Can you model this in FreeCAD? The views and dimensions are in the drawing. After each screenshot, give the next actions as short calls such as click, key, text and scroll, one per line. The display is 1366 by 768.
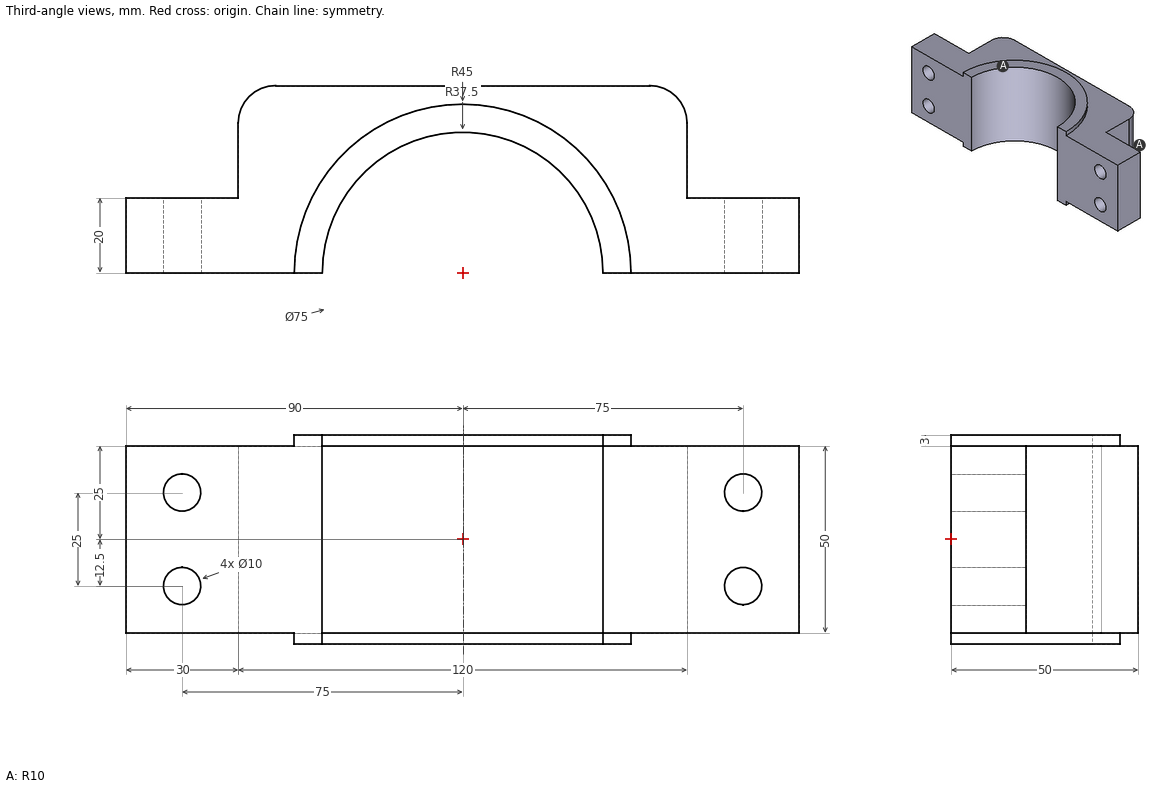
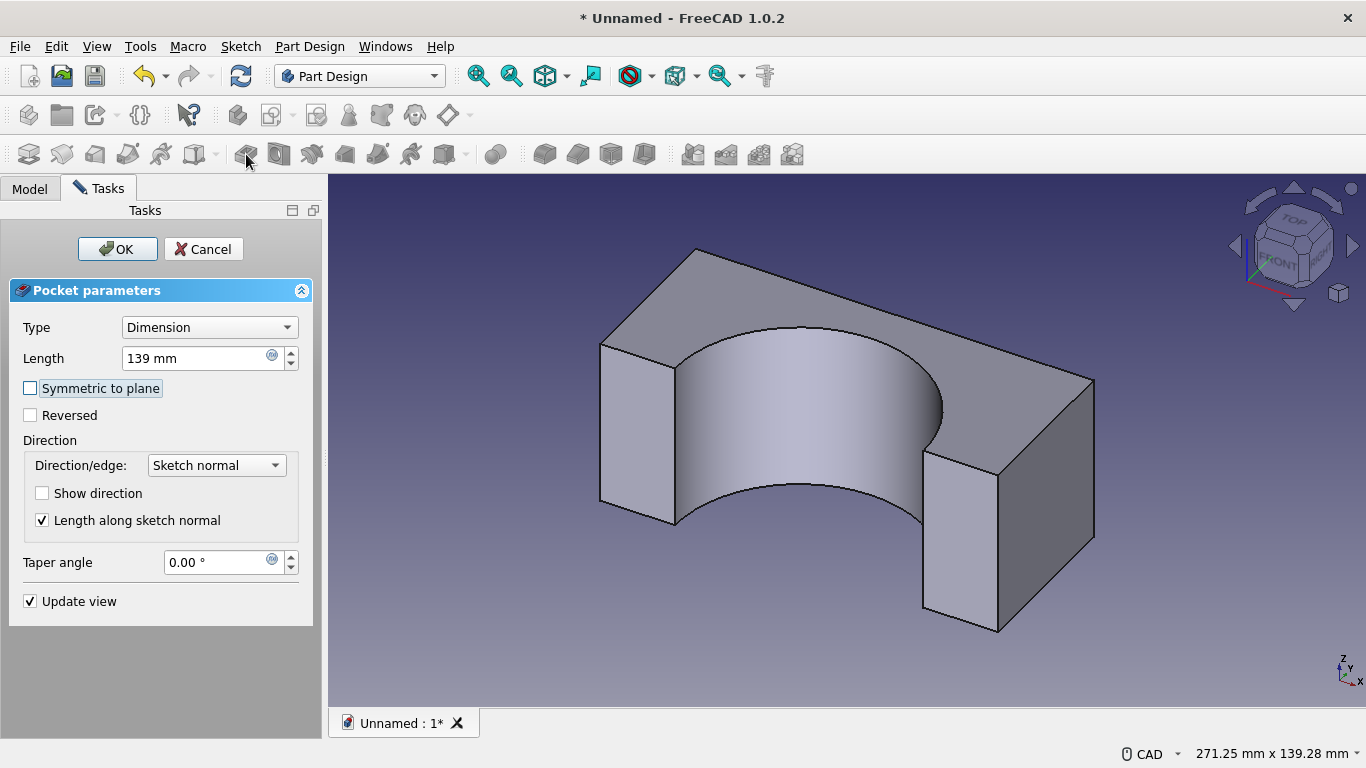
click(118, 249)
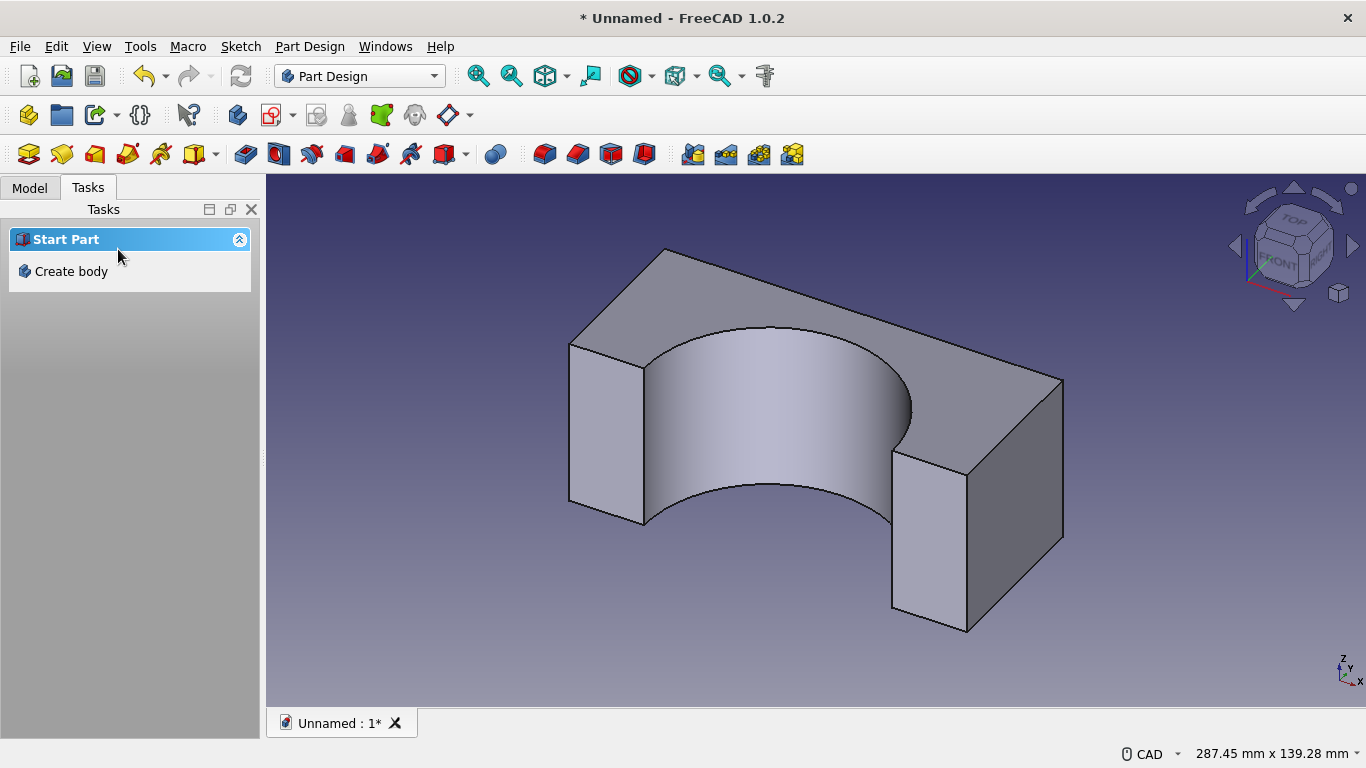
key(0)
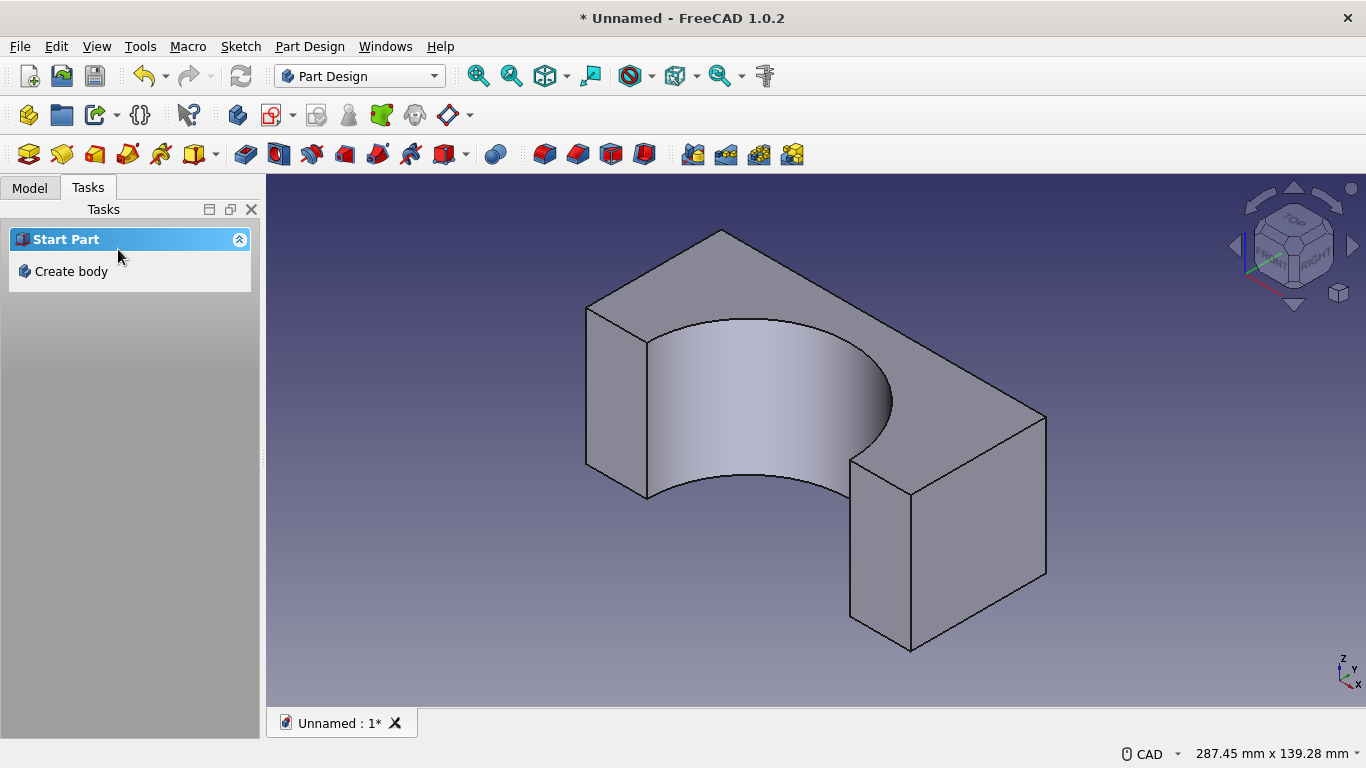
key(2)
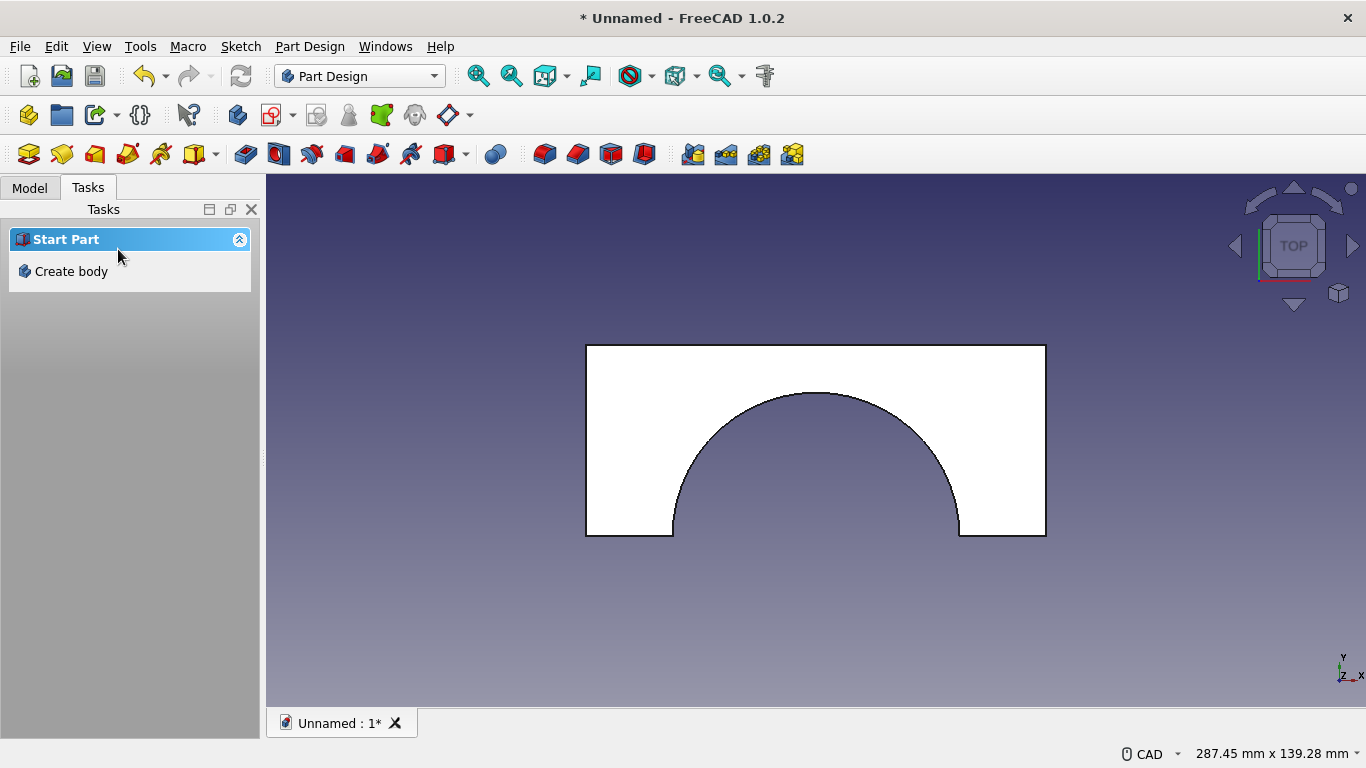
key(v)
key(f)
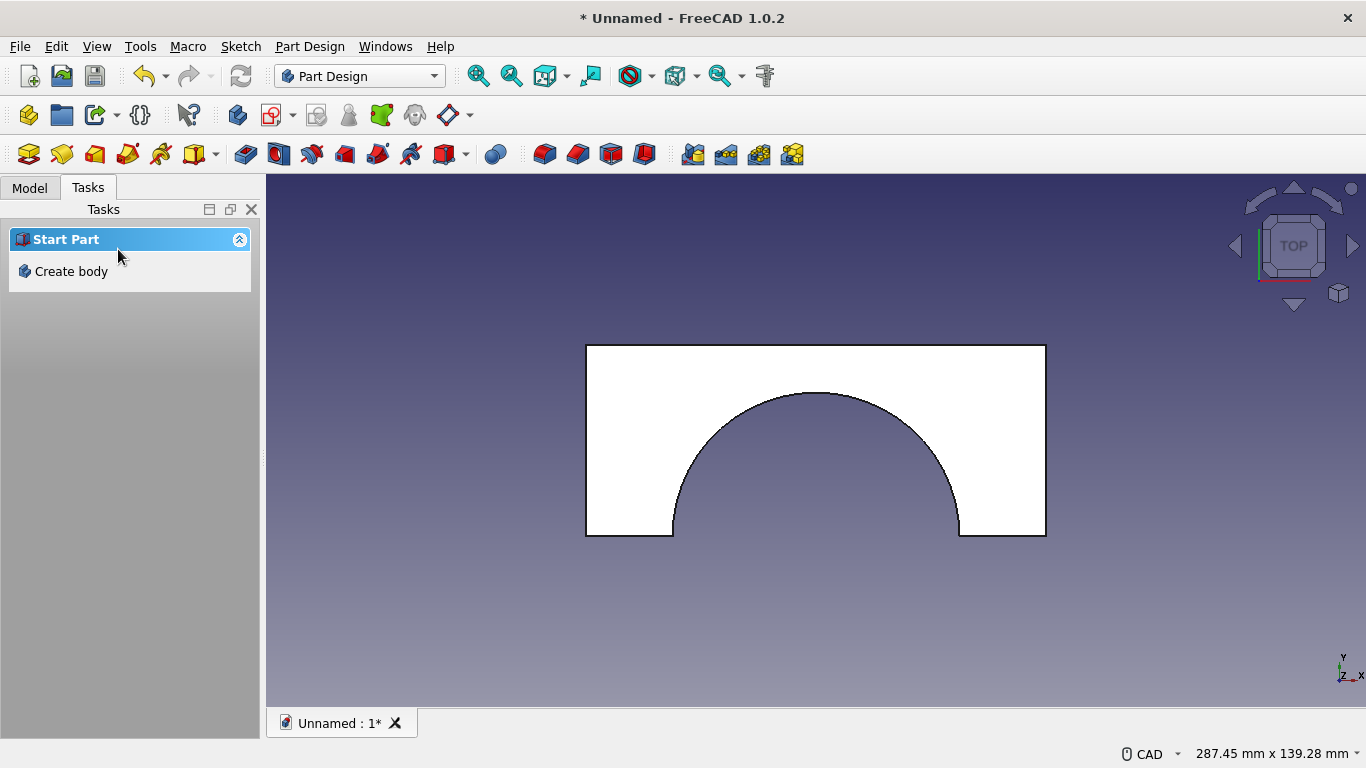
key(1)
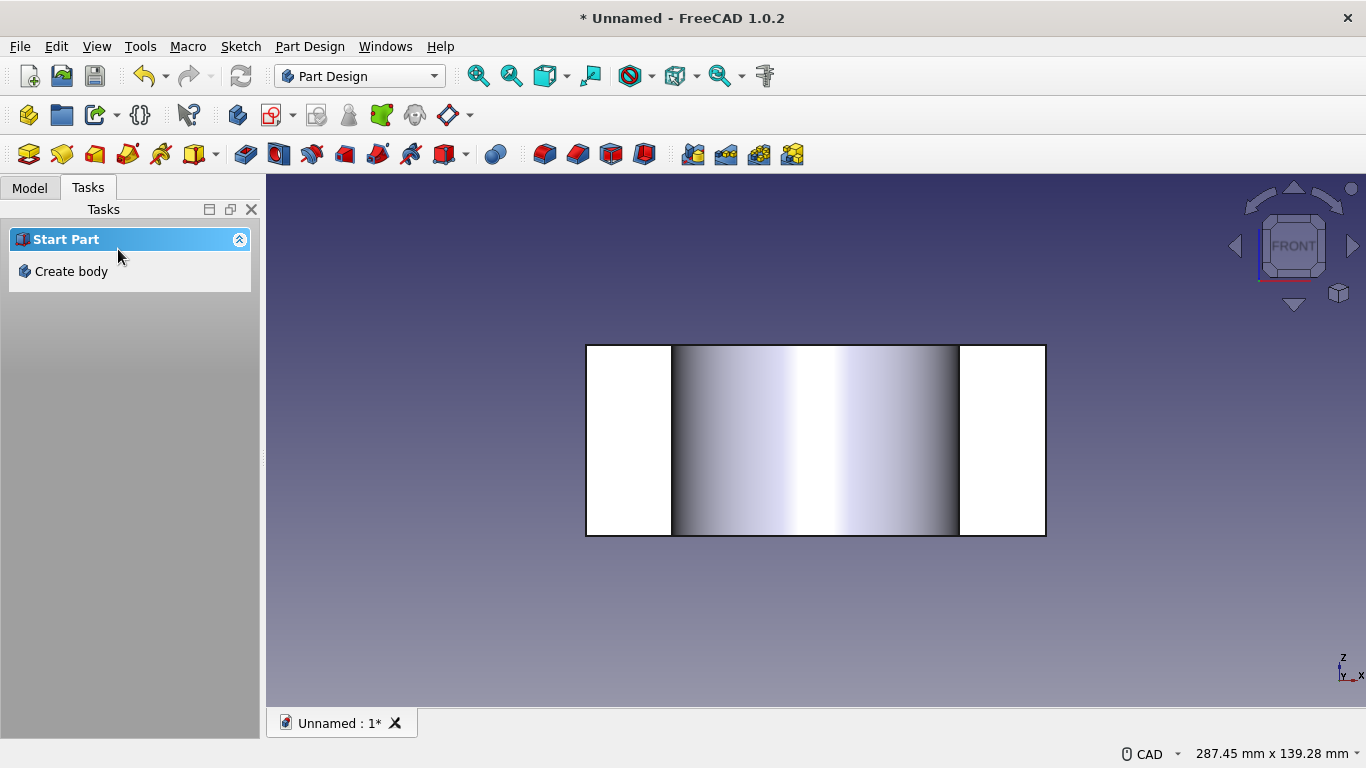
click(479, 76)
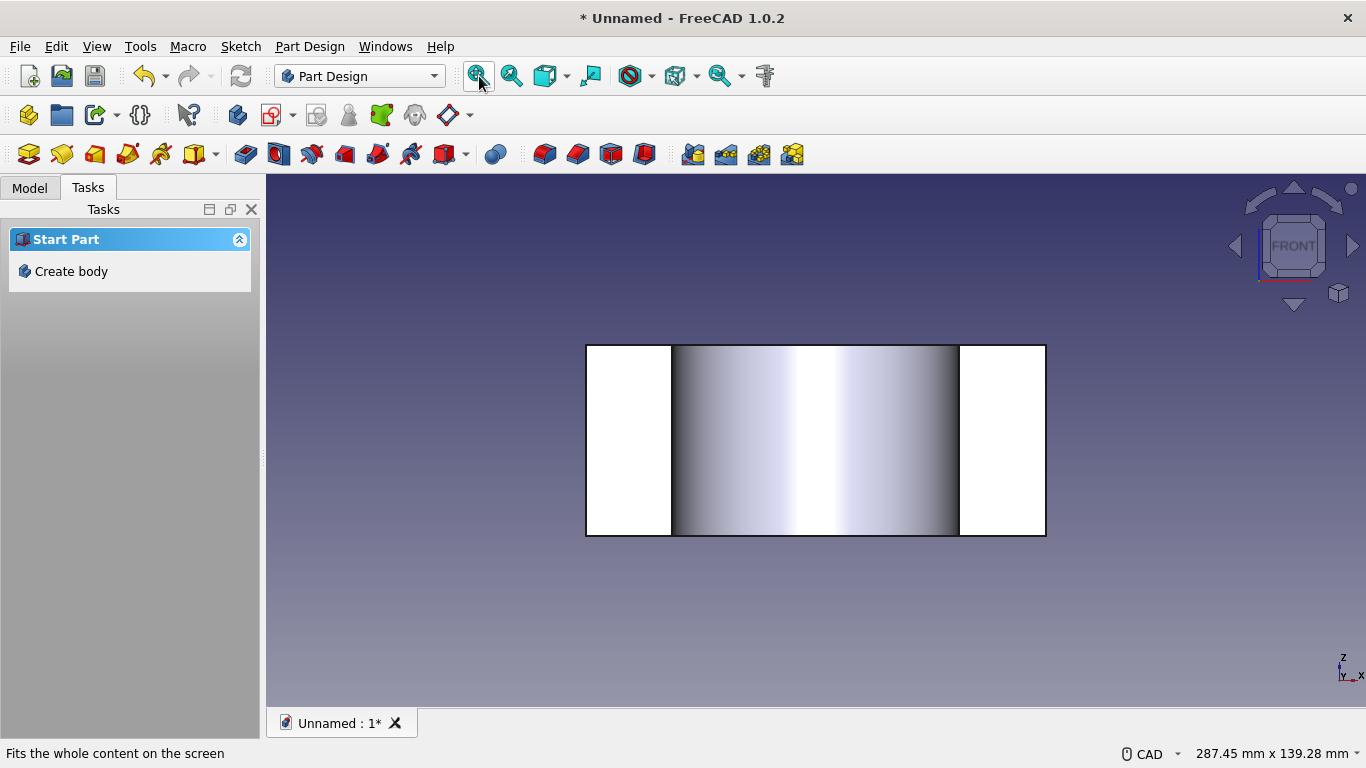
key(3)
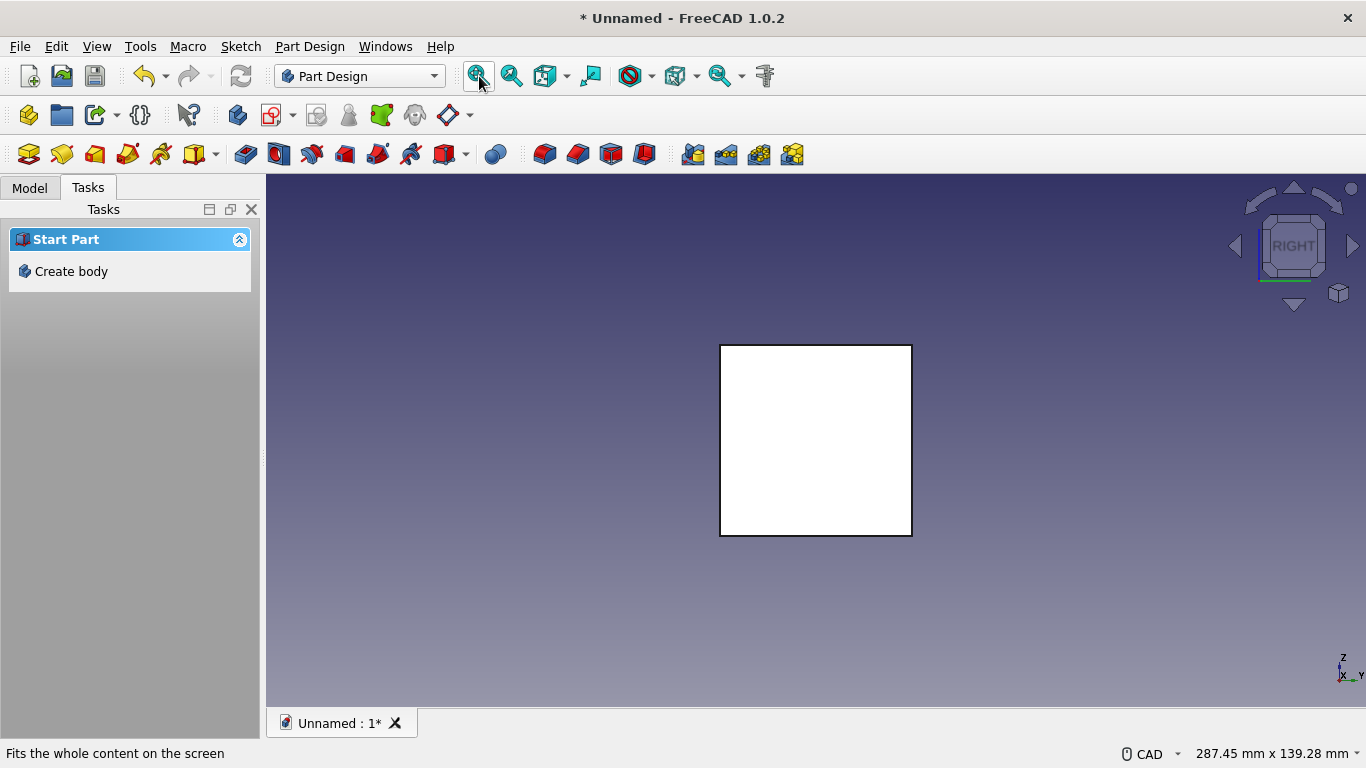
key(v)
key(f)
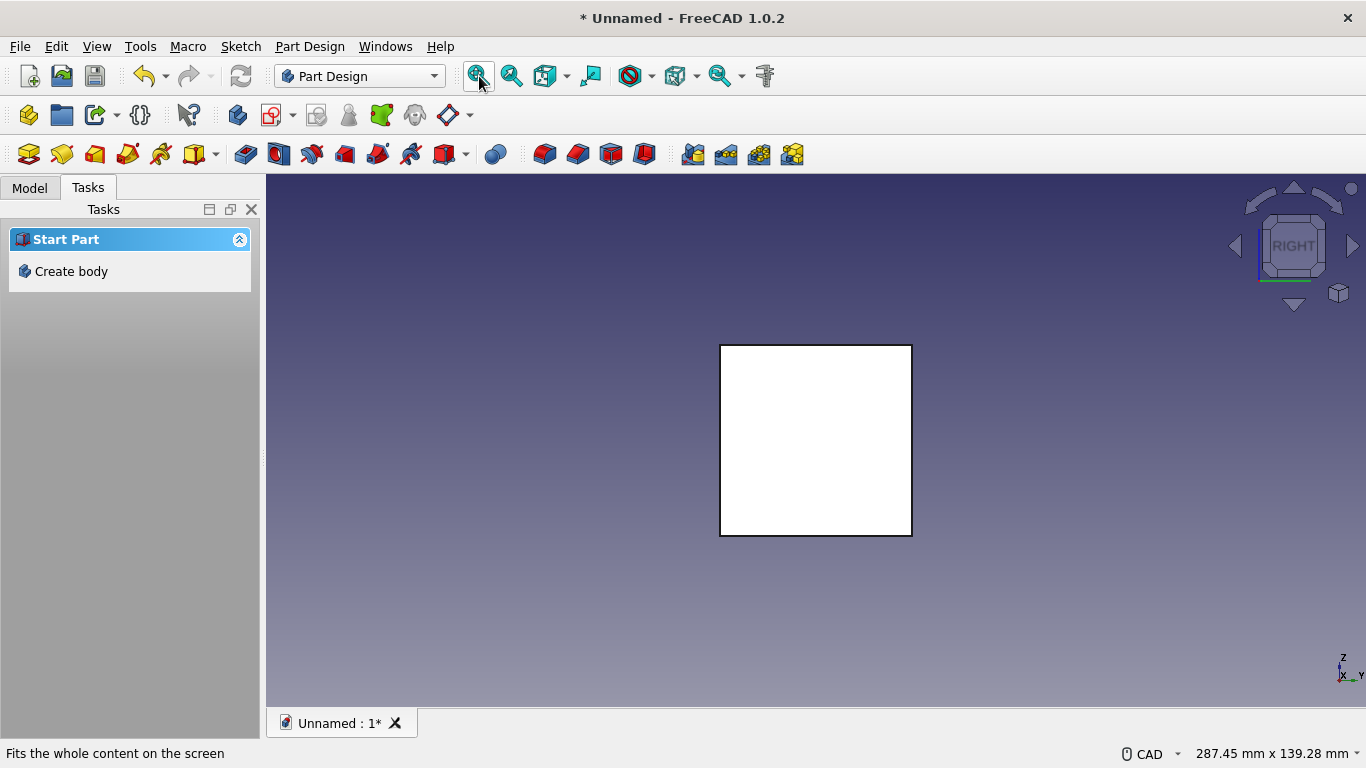
click(912, 440)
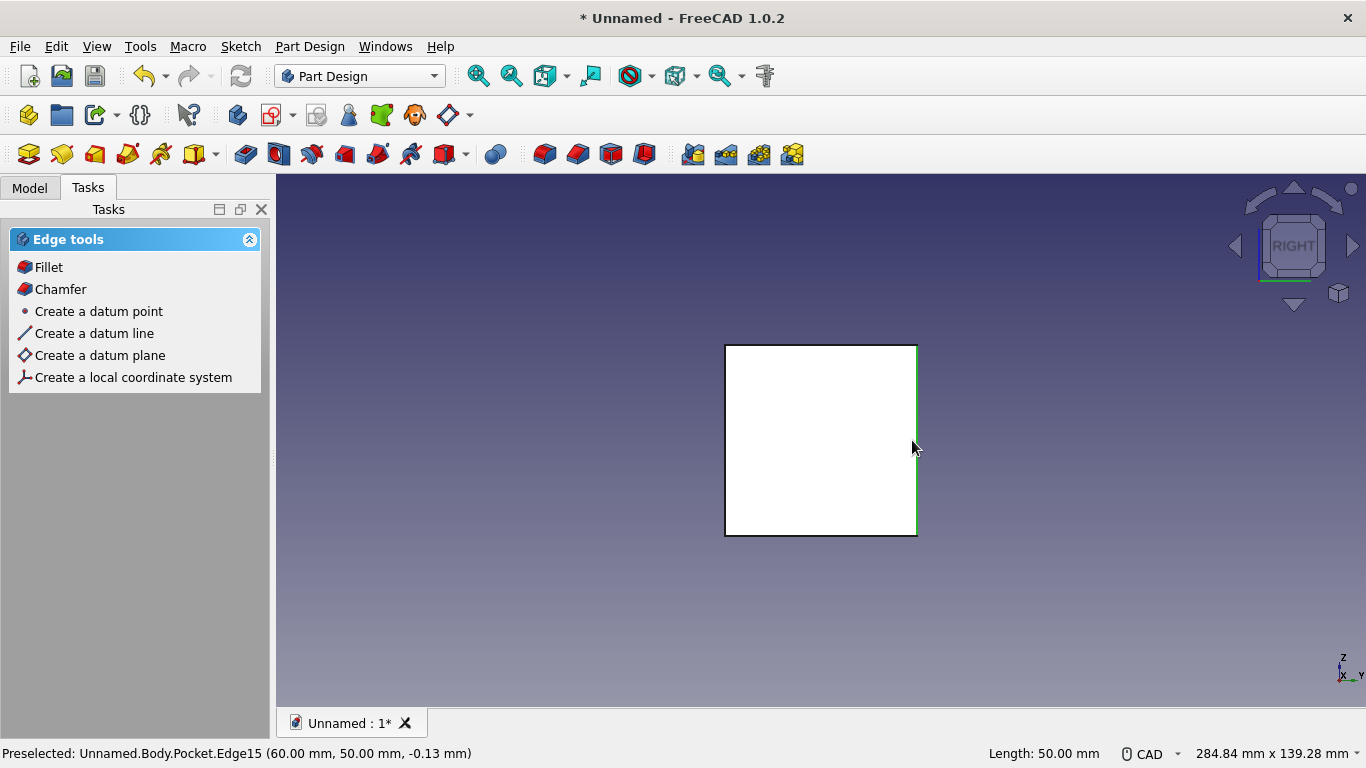
key(5)